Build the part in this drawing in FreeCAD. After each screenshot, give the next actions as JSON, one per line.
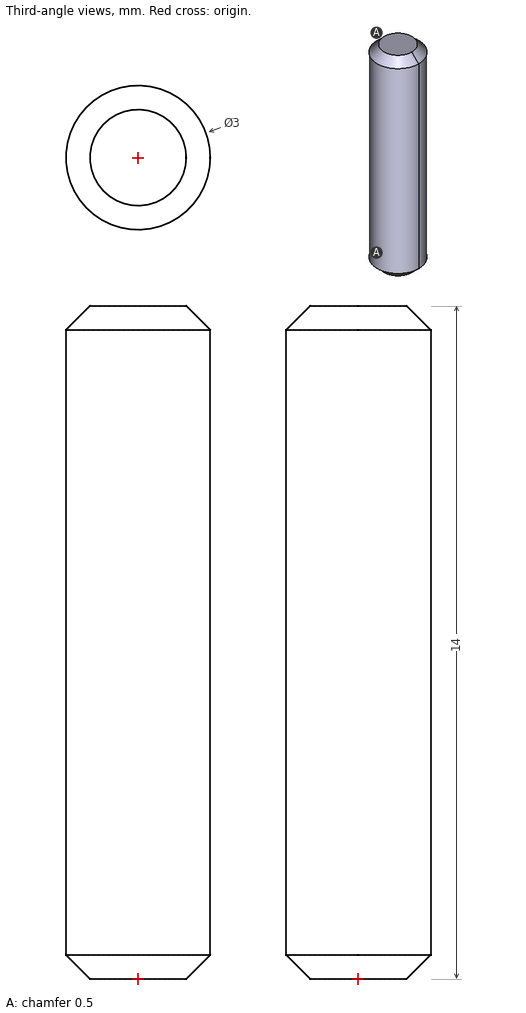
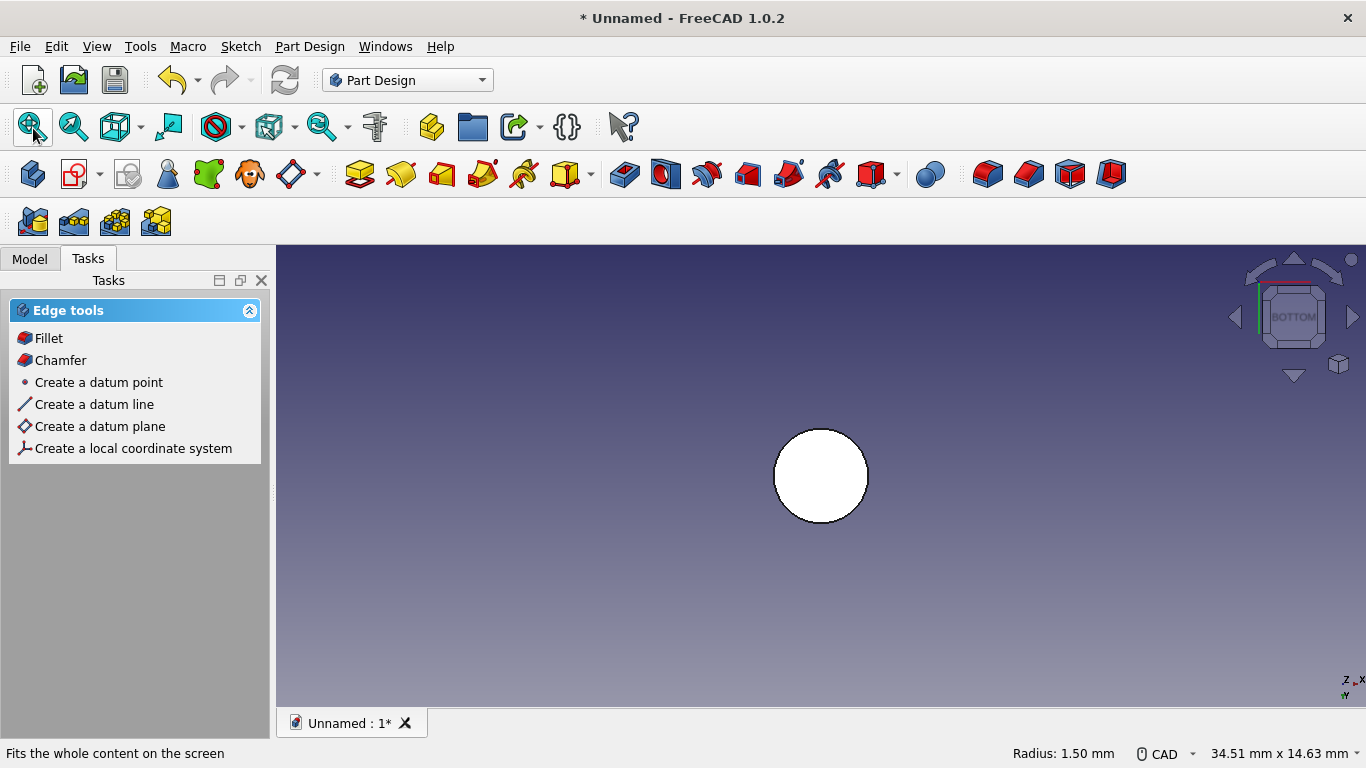
{"action": "left_click", "coordinate": [33, 128]}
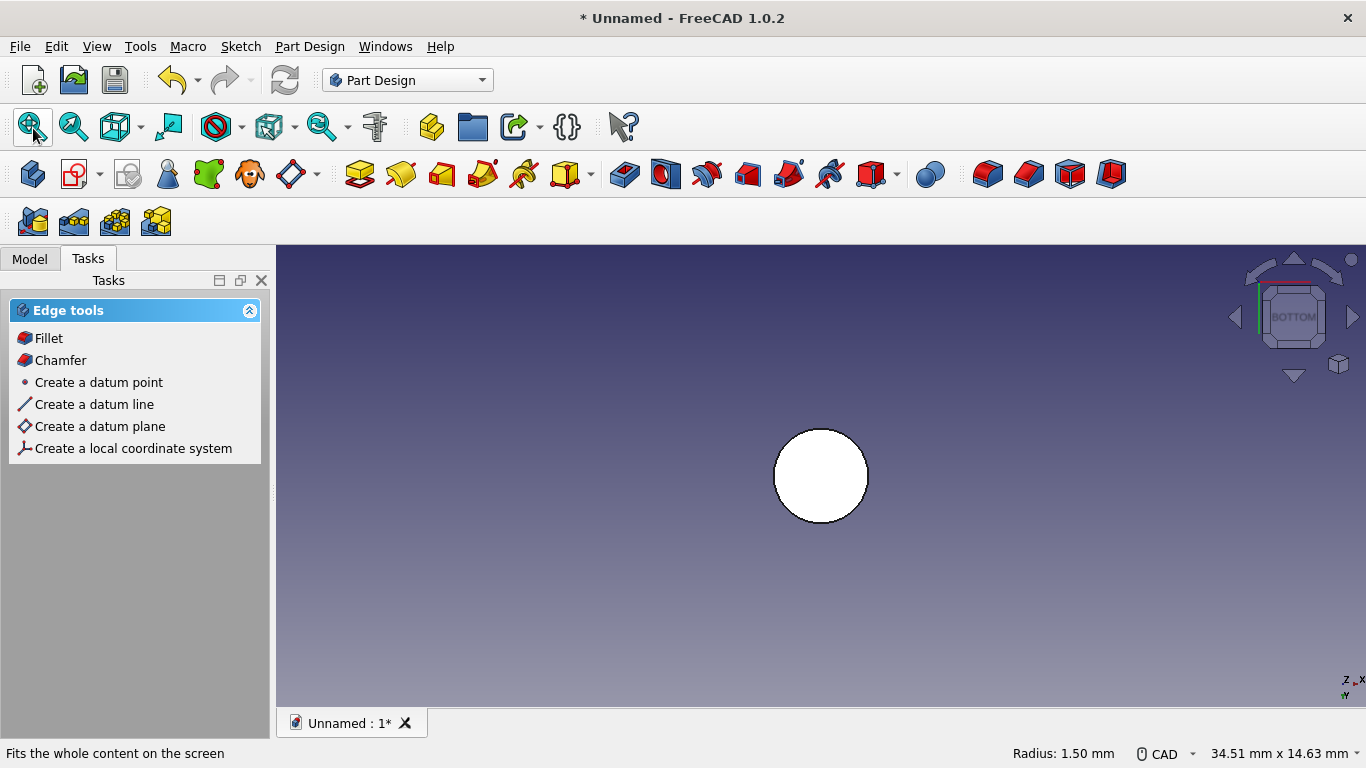
{"action": "left_click", "coordinate": [774, 475], "text": "ctrl"}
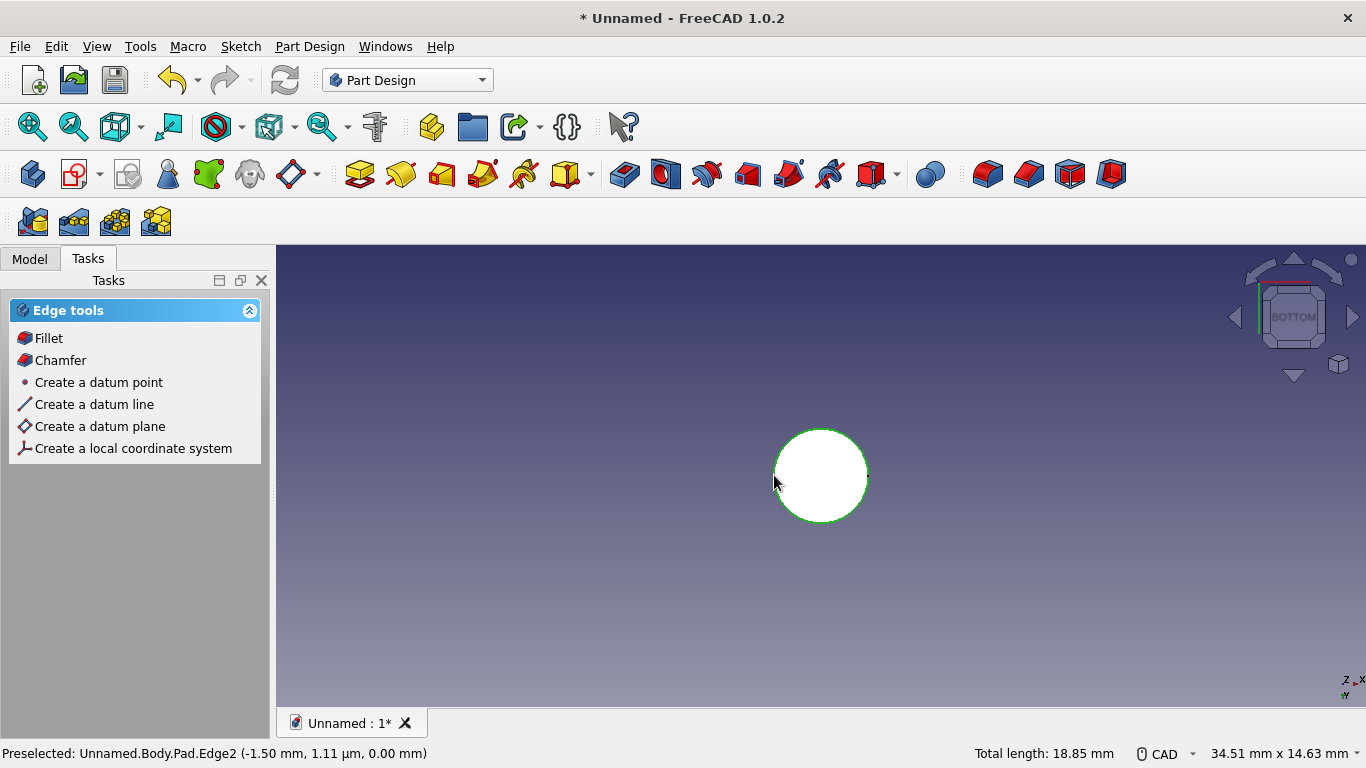
{"action": "left_click", "coordinate": [1029, 174]}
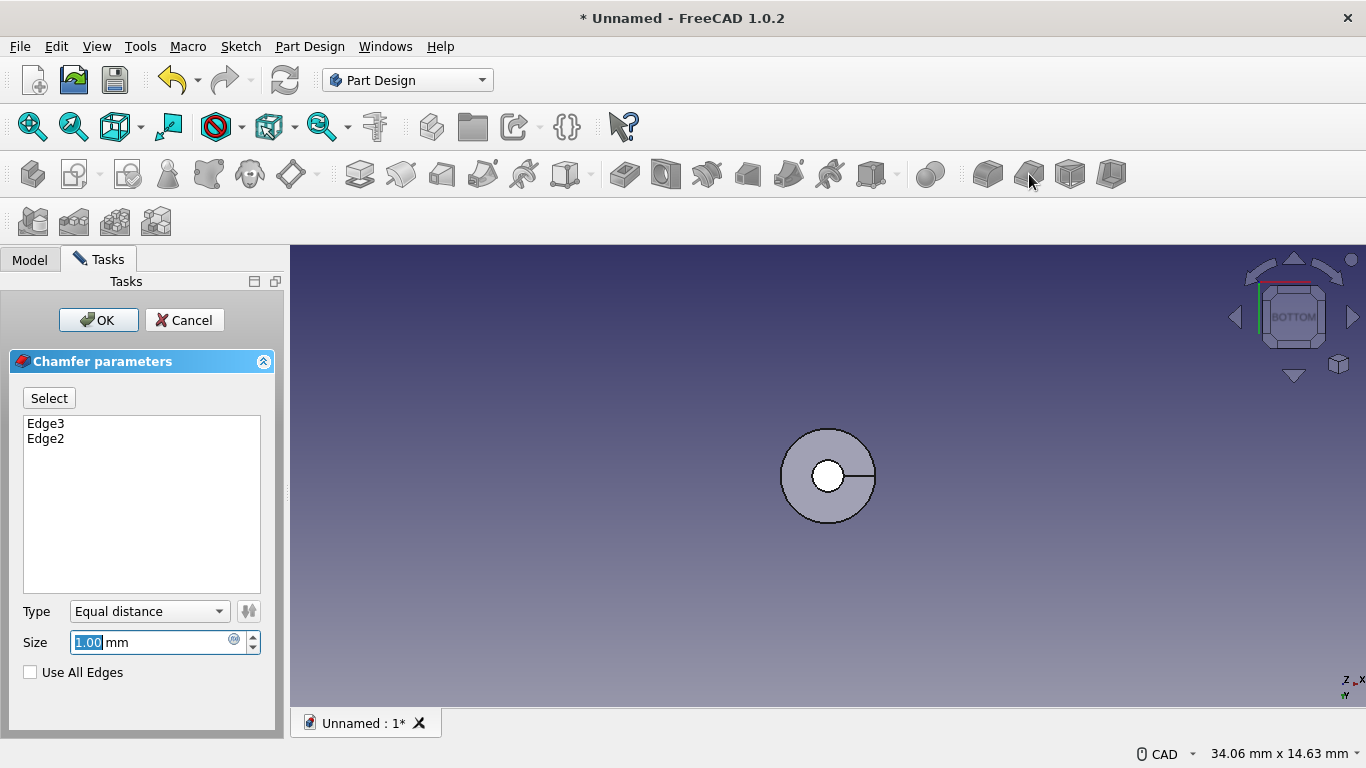
{"action": "type", "text": "0.5"}
{"action": "key", "text": "Tab"}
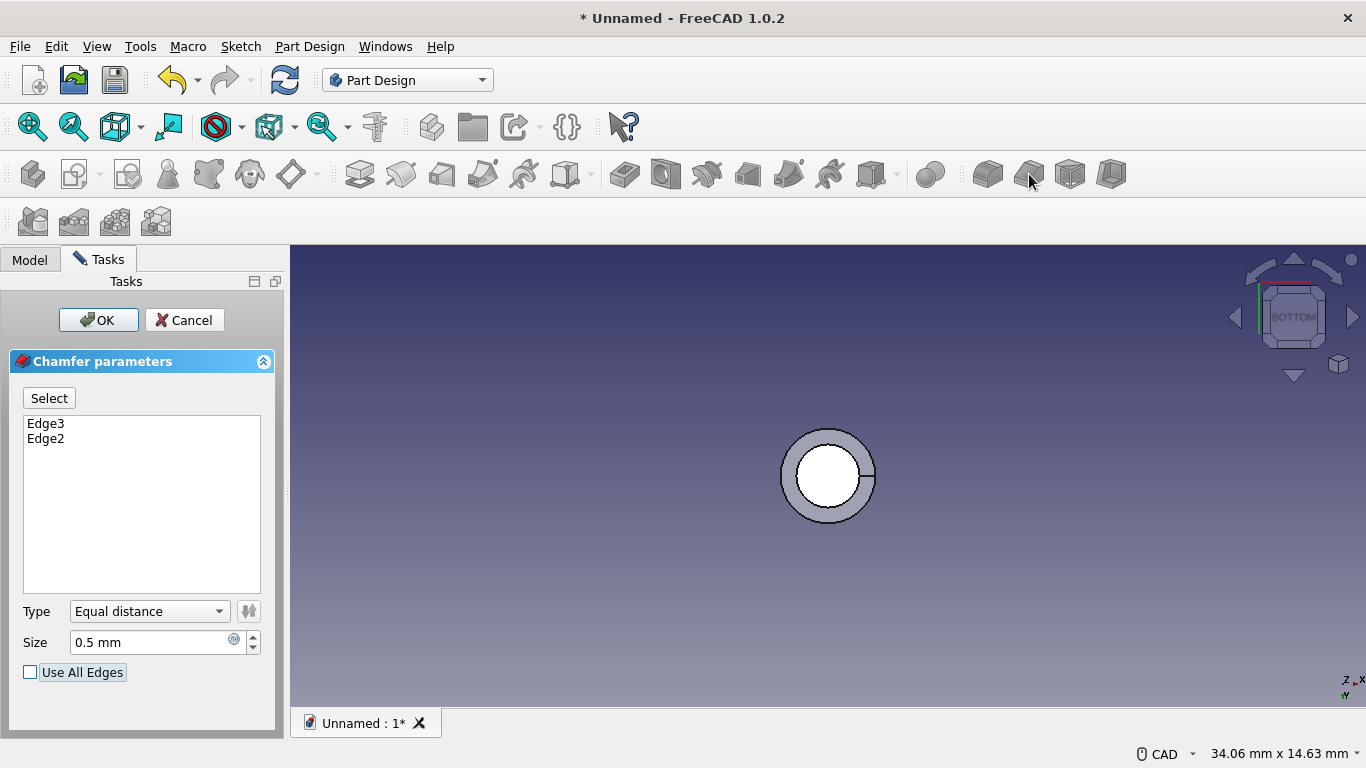
{"action": "left_click", "coordinate": [99, 320]}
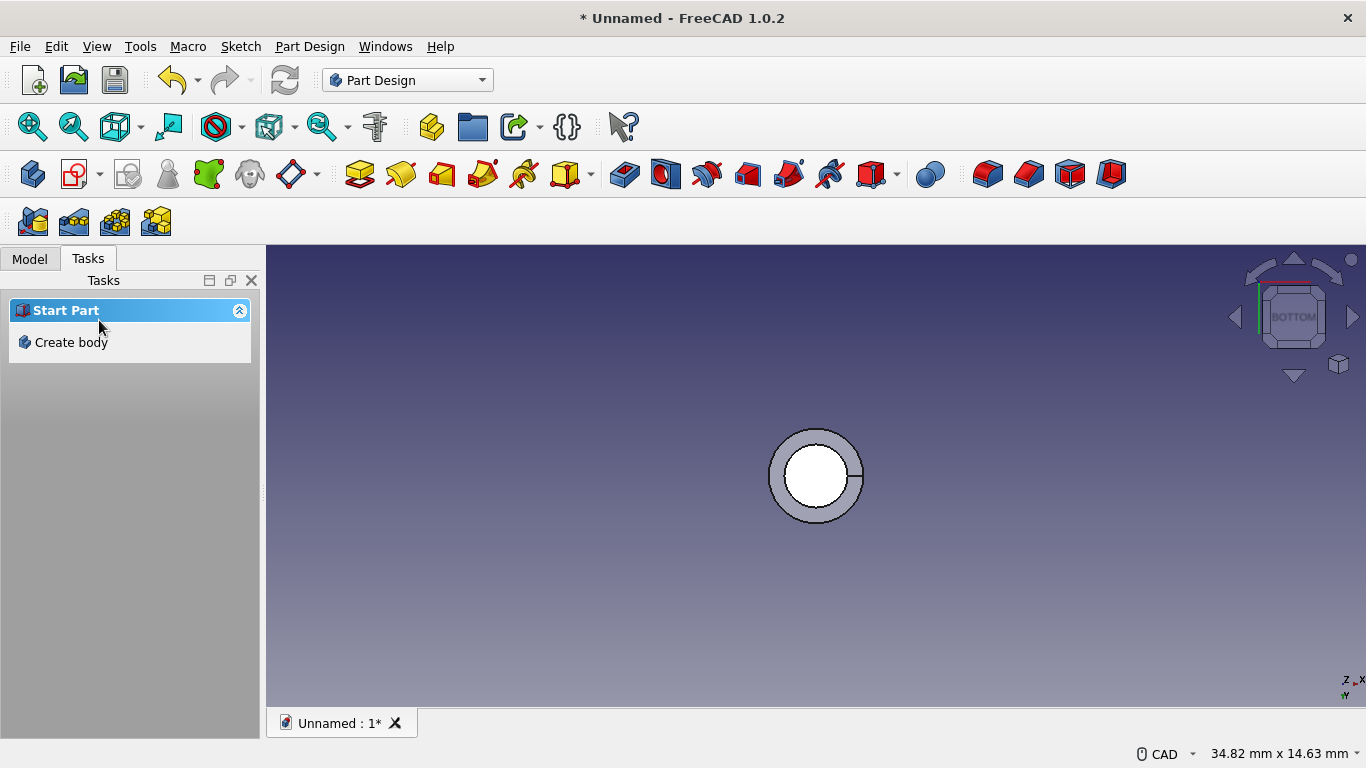
{"action": "key", "text": "0"}